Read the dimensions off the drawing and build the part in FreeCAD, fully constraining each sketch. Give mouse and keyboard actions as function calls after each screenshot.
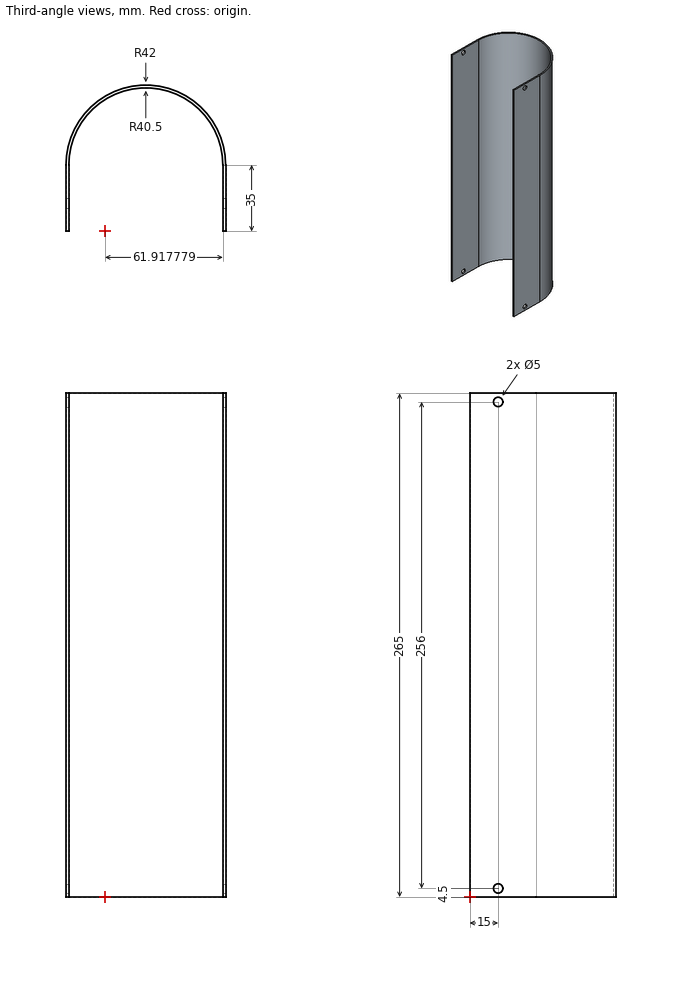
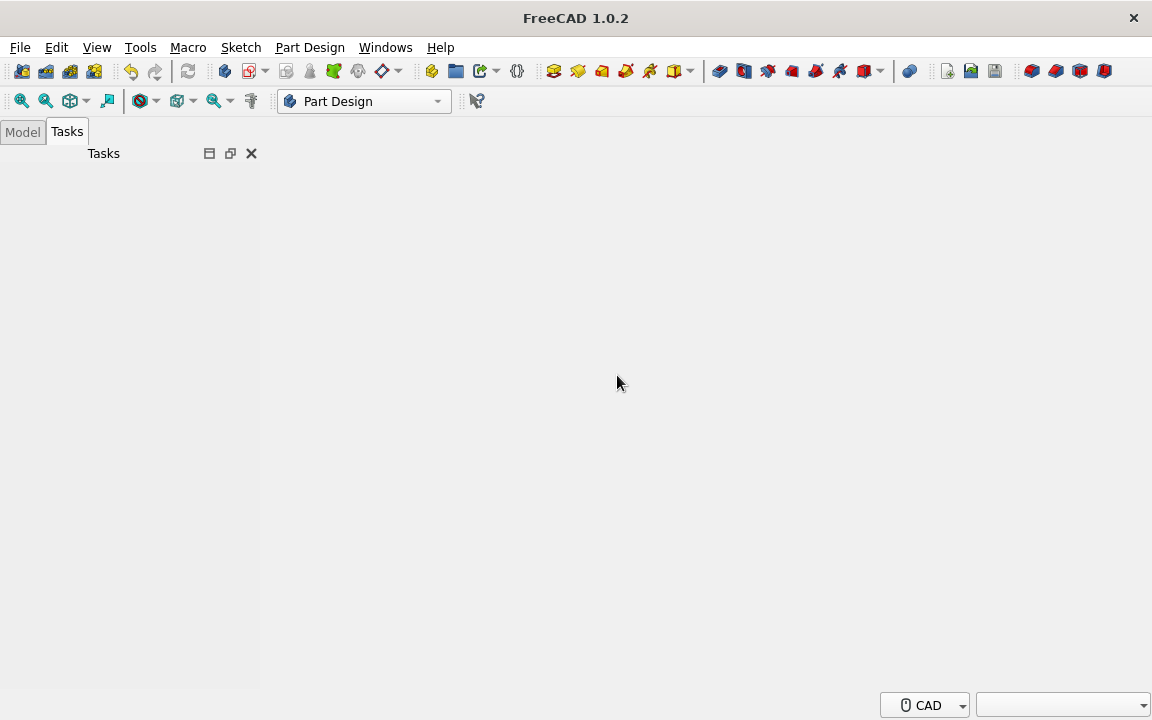
click(948, 72)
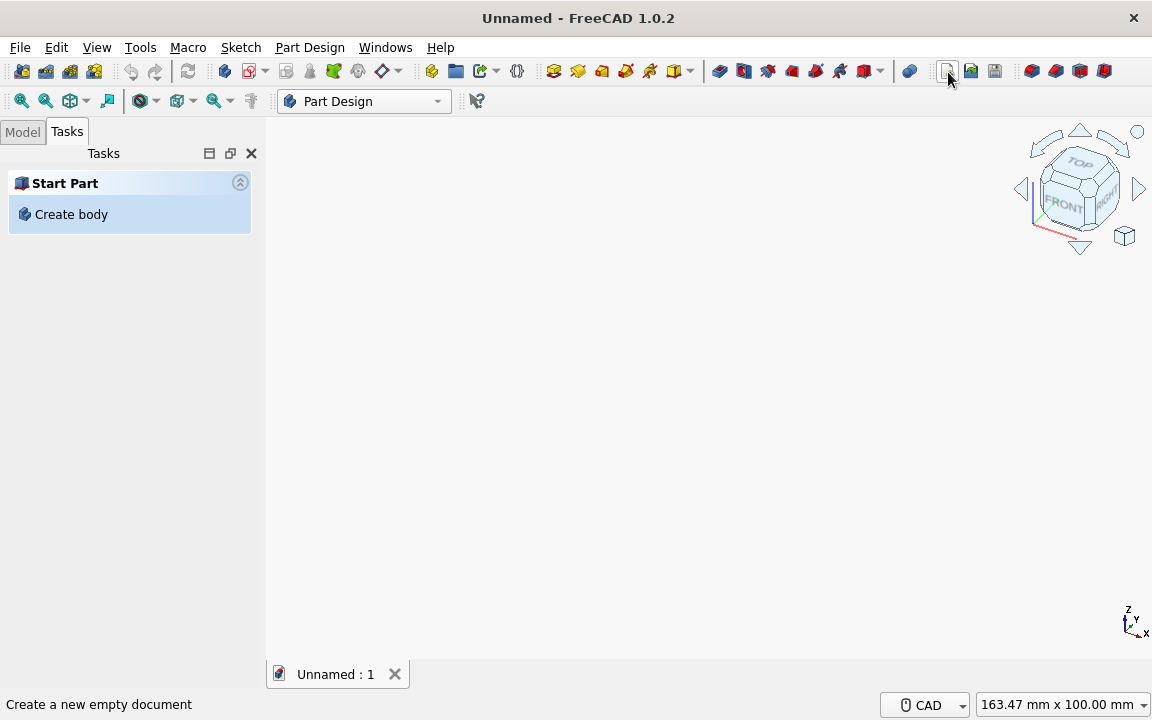
click(250, 72)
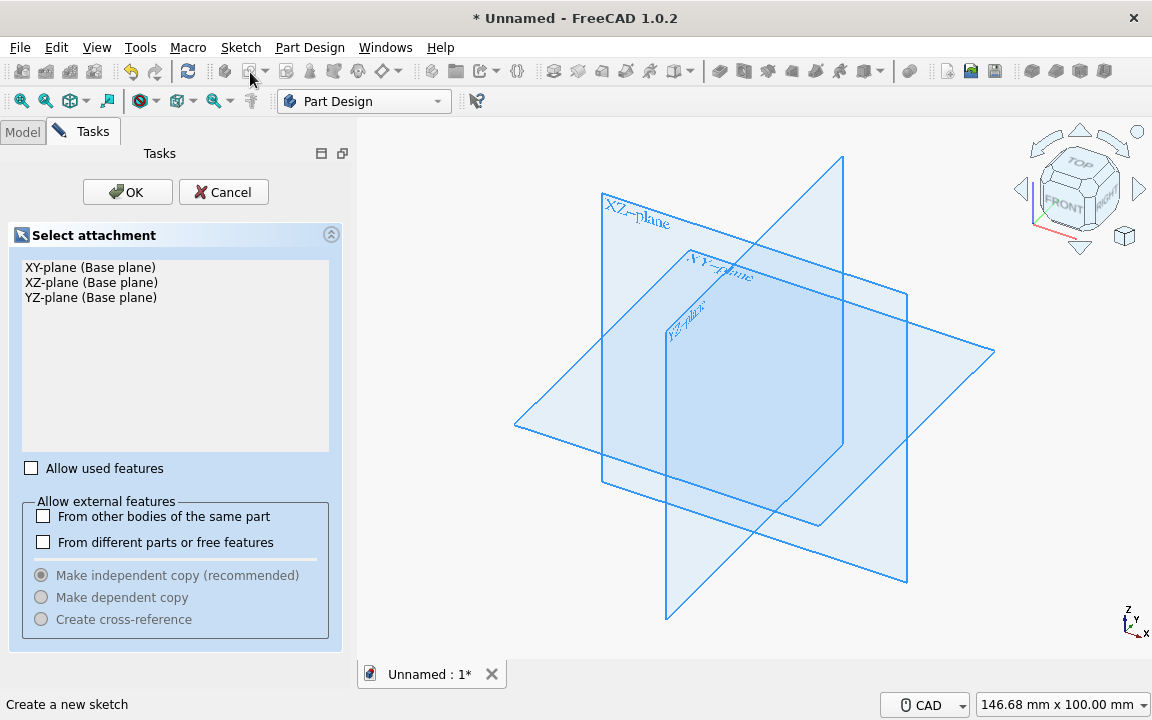
click(82, 268)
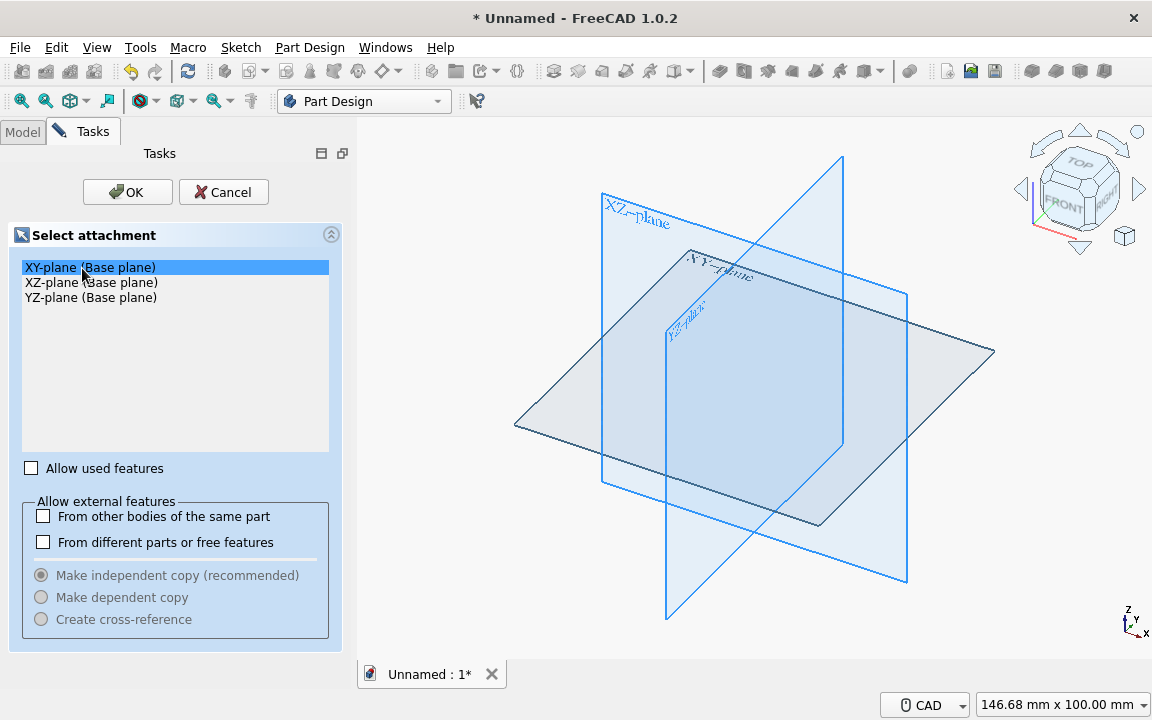
click(128, 192)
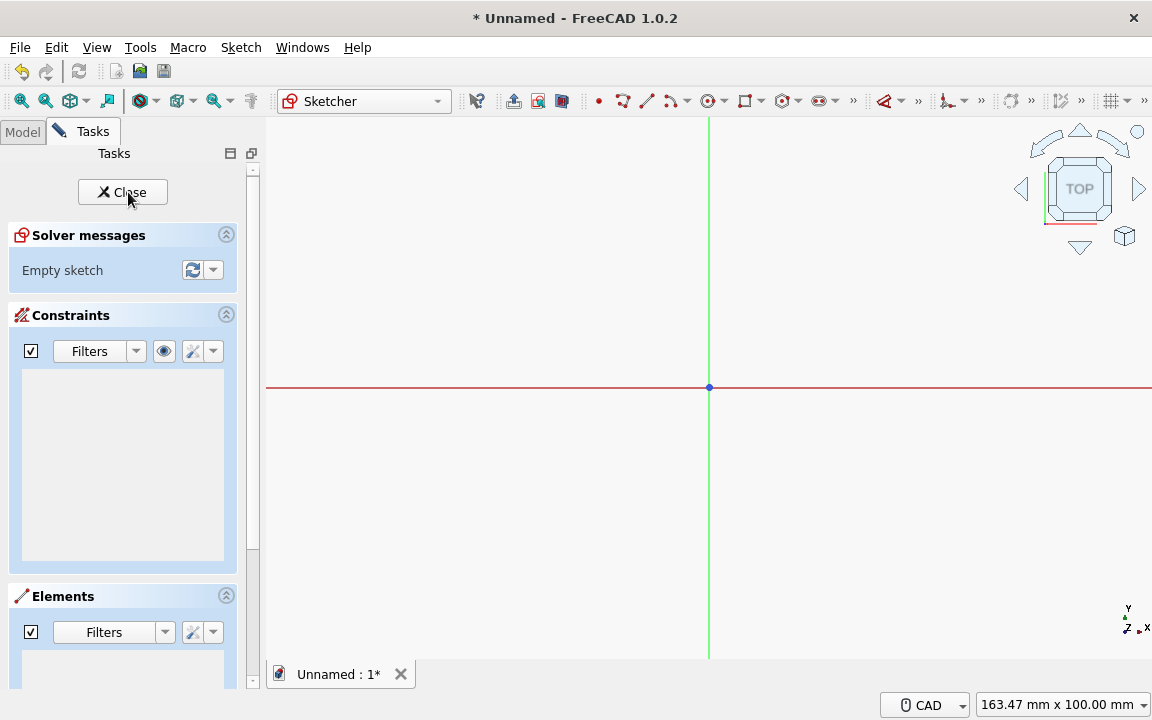
scroll(294, 631, down, 2)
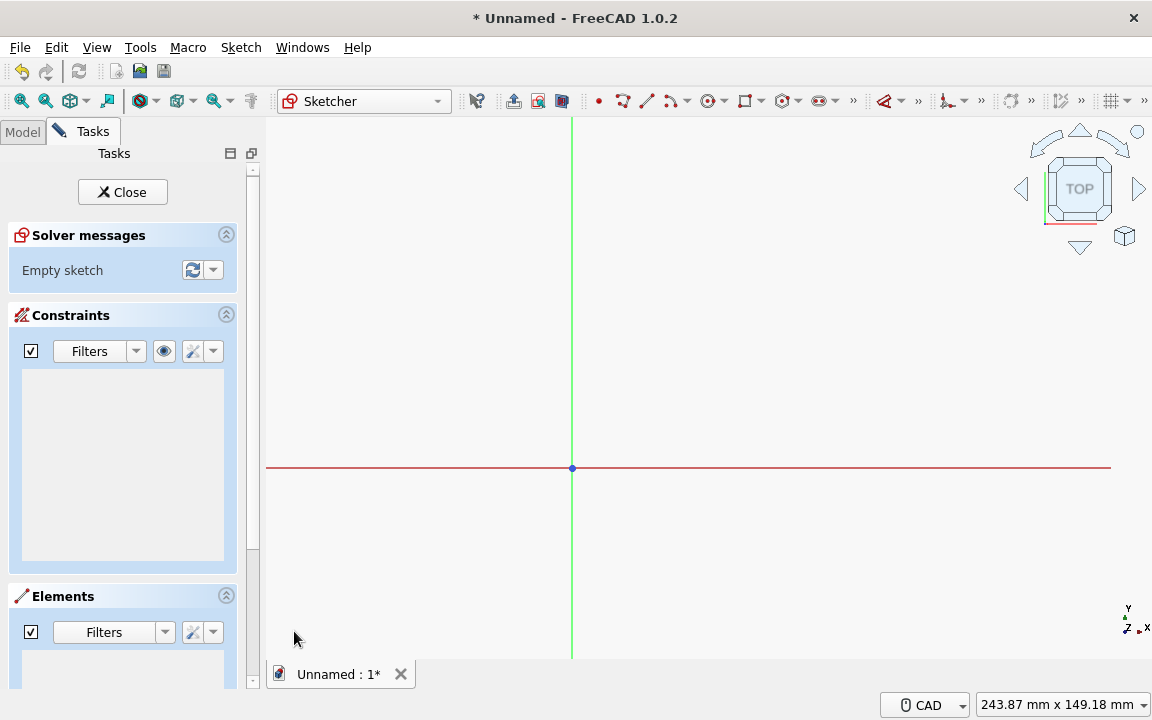
click(624, 102)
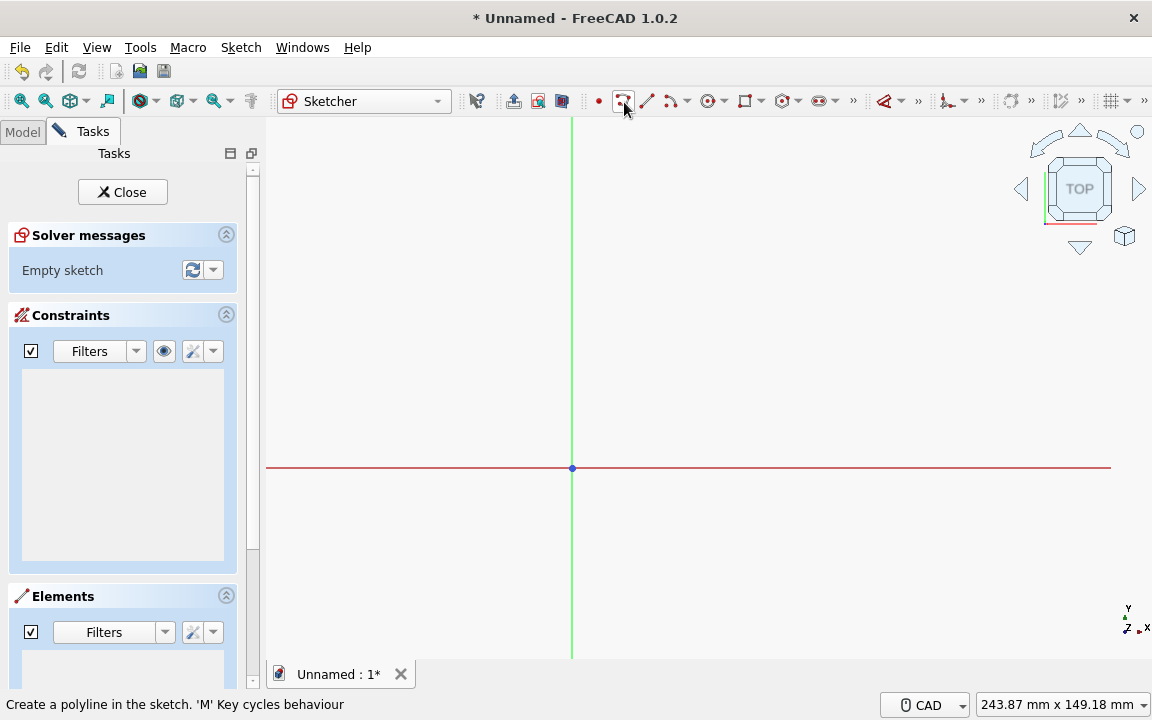
click(797, 341)
click(797, 468)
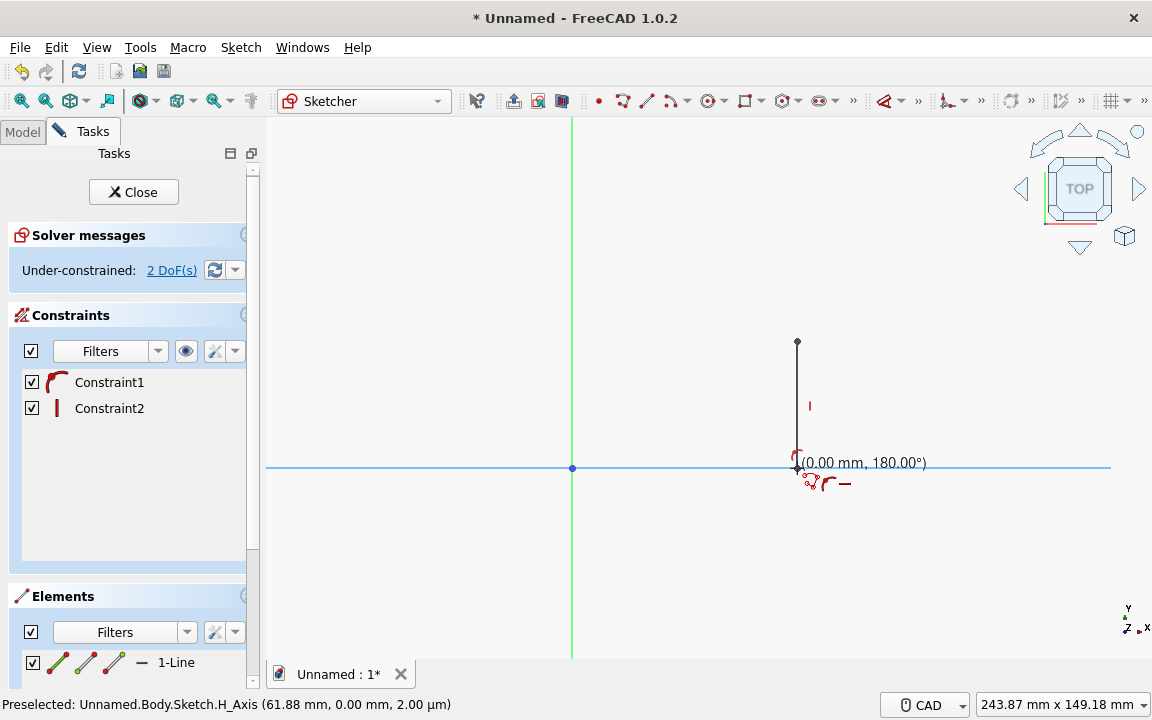
scroll(803, 468, up, 6)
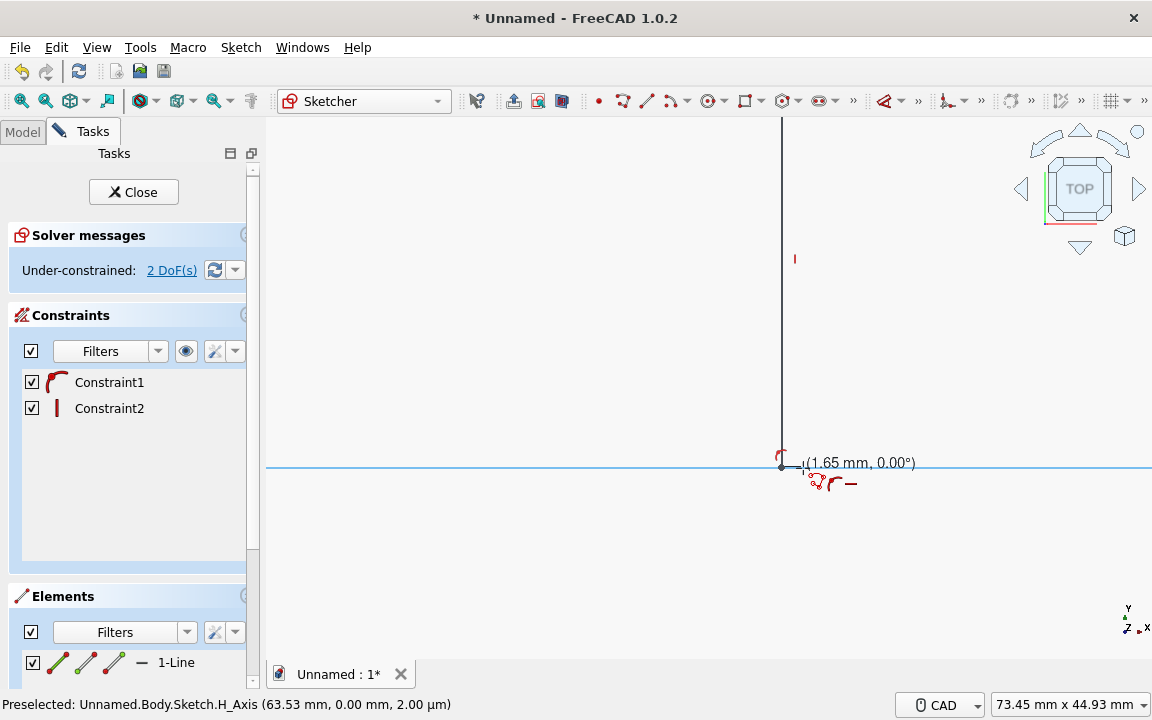
click(800, 459)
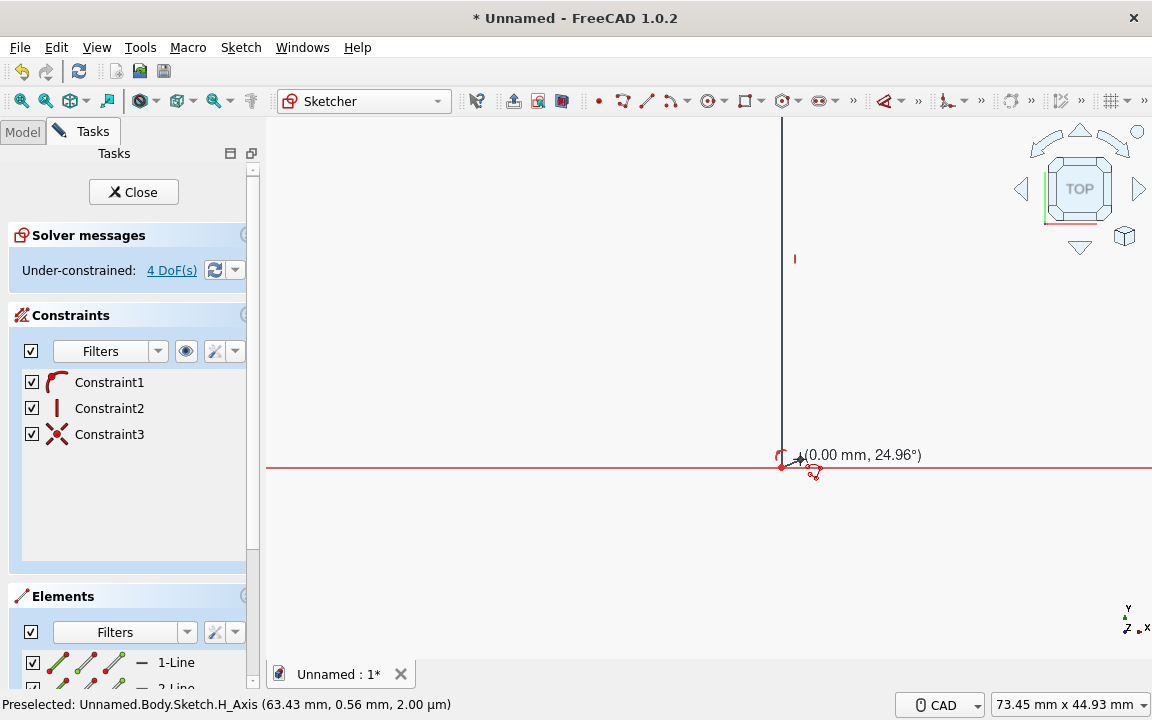
scroll(842, 612, down, 5)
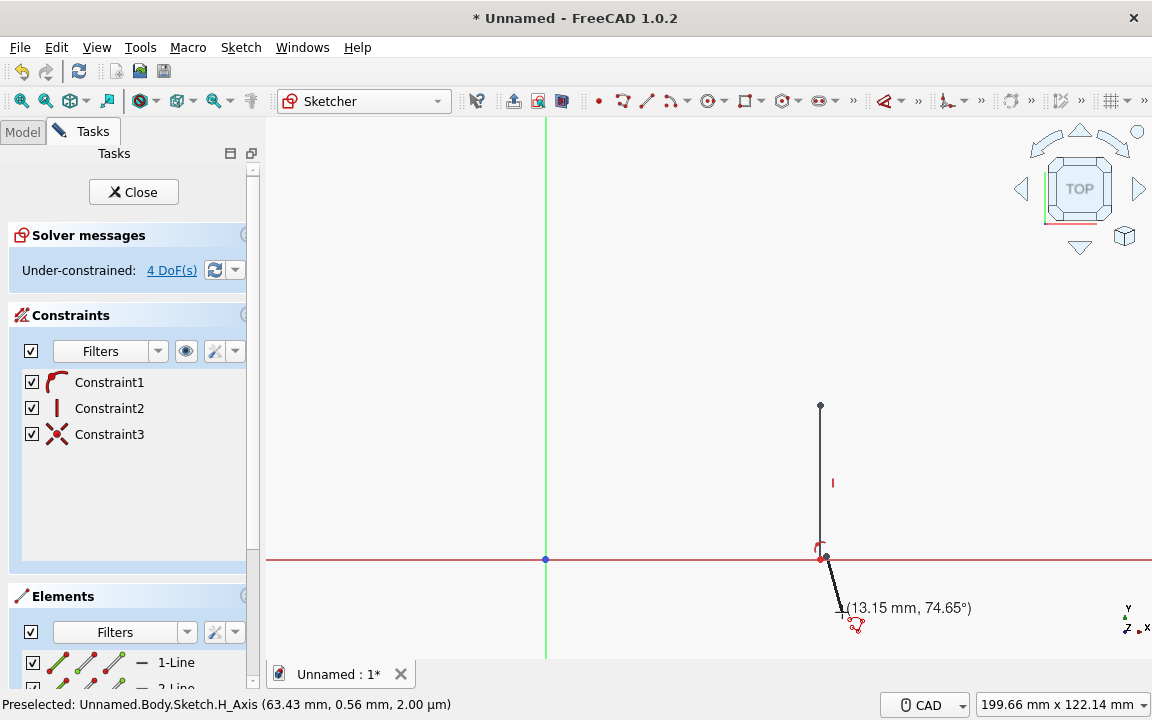
scroll(827, 404, up, 5)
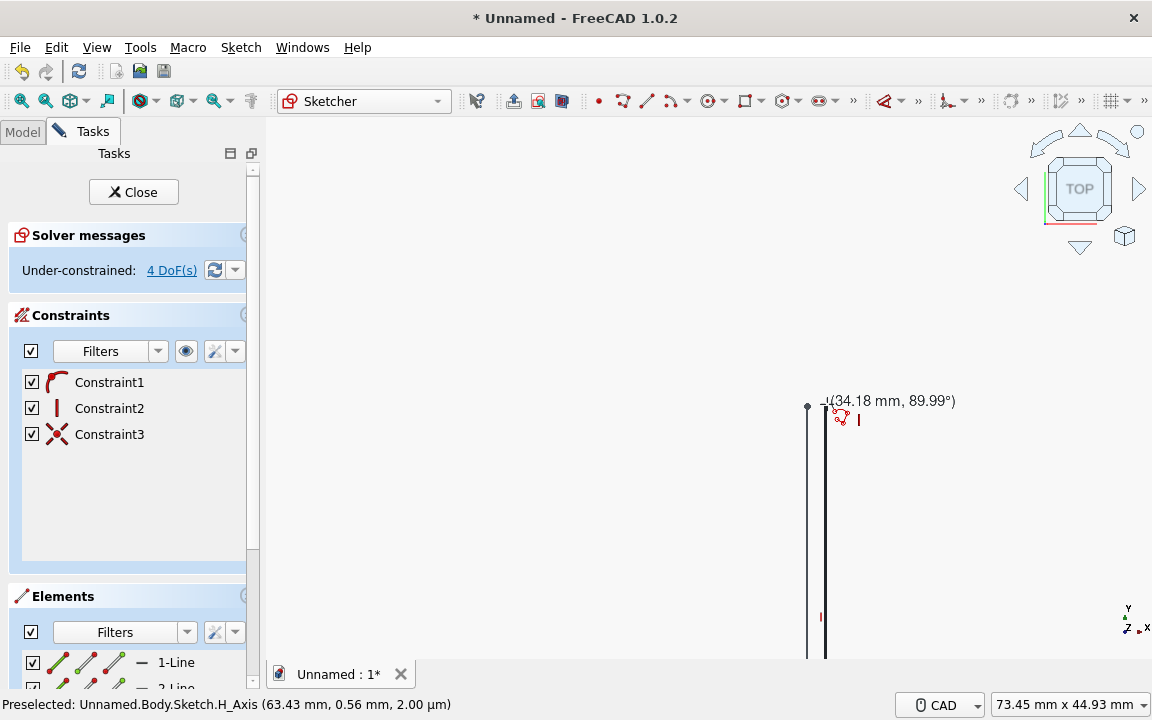
click(826, 404)
right_click(826, 404)